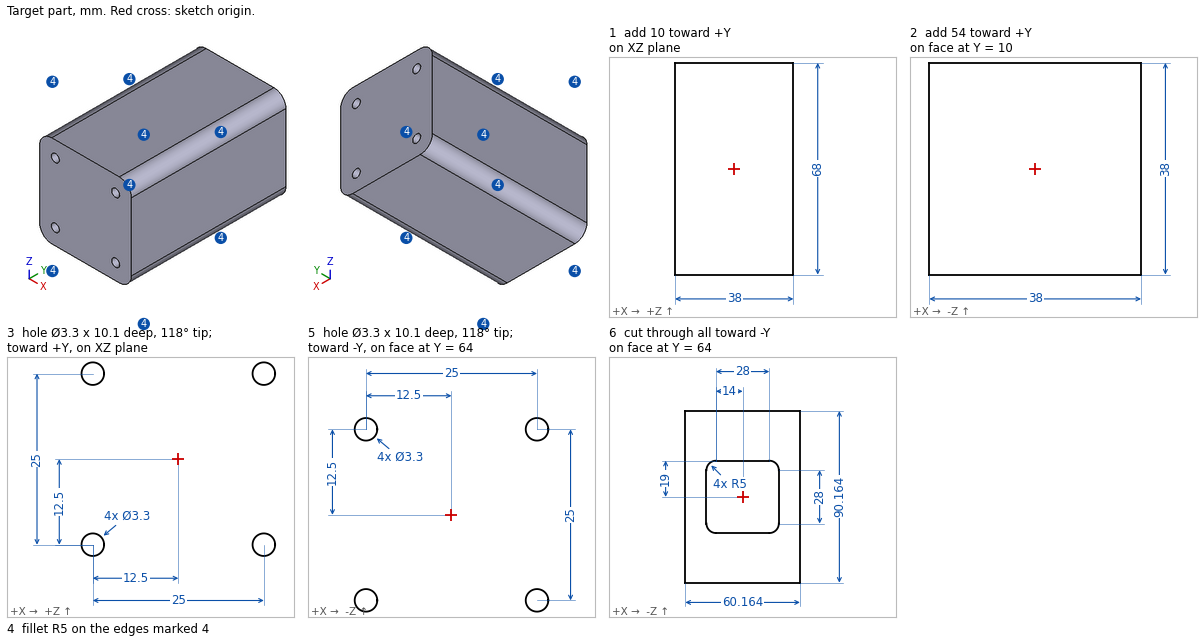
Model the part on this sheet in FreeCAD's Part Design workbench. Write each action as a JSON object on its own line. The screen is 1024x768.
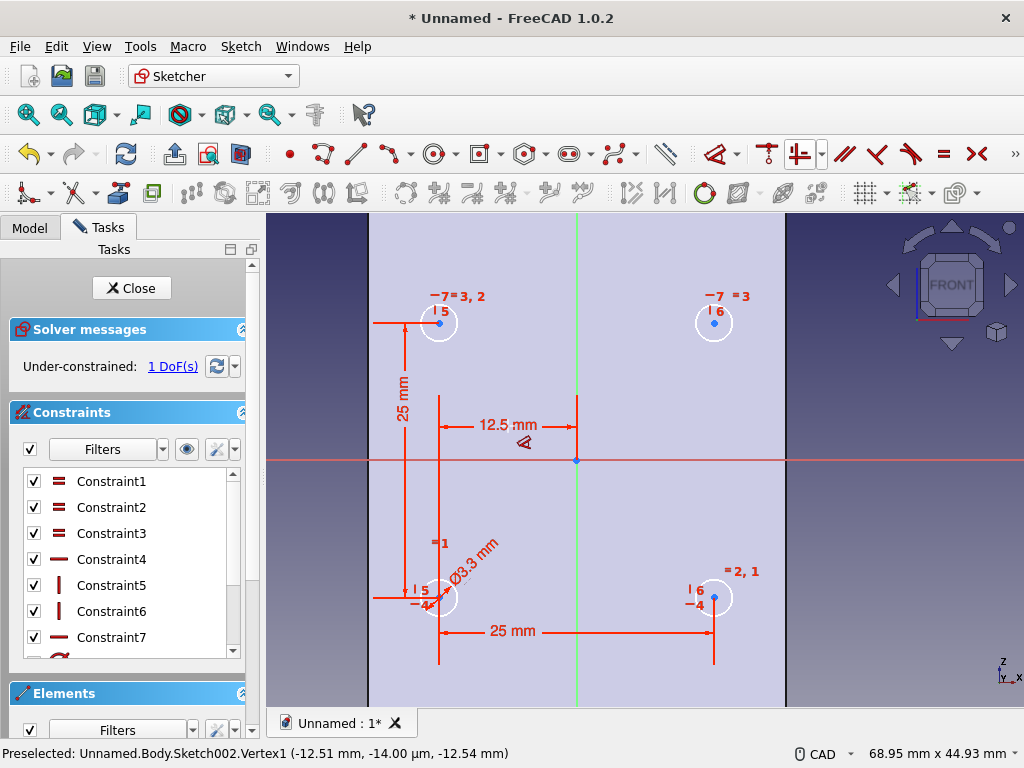
{"action": "left_click", "coordinate": [439, 598]}
{"action": "left_click", "coordinate": [405, 529]}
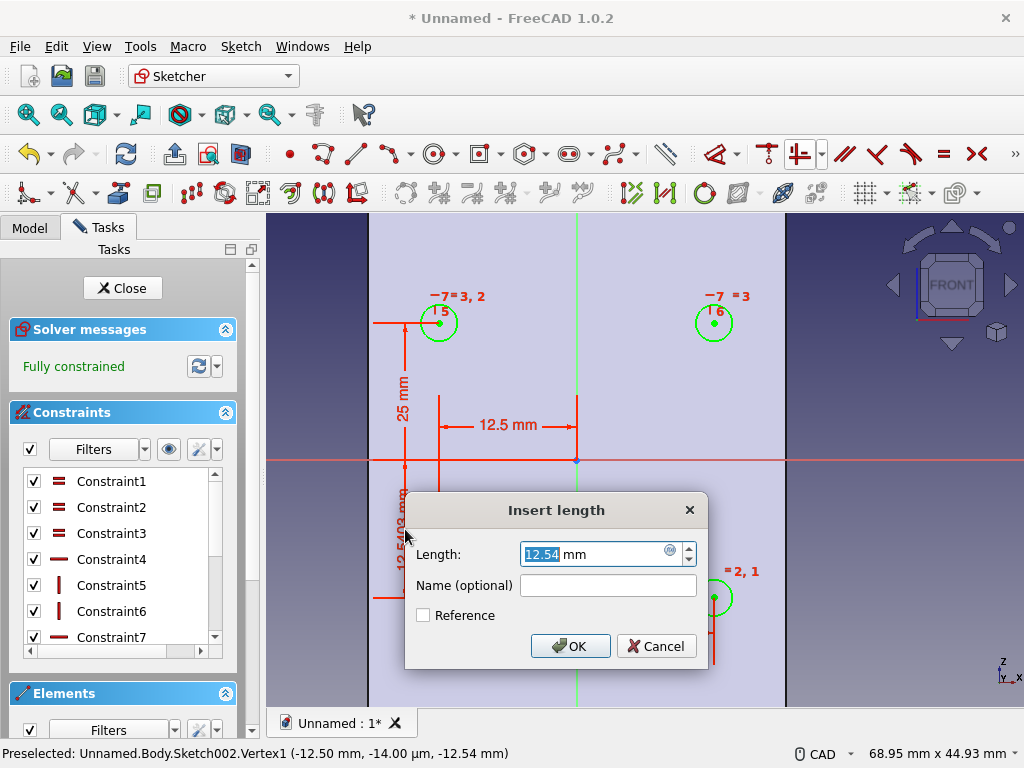
{"action": "type", "text": "12.5"}
{"action": "key", "text": "Return"}
{"action": "key", "text": "Escape"}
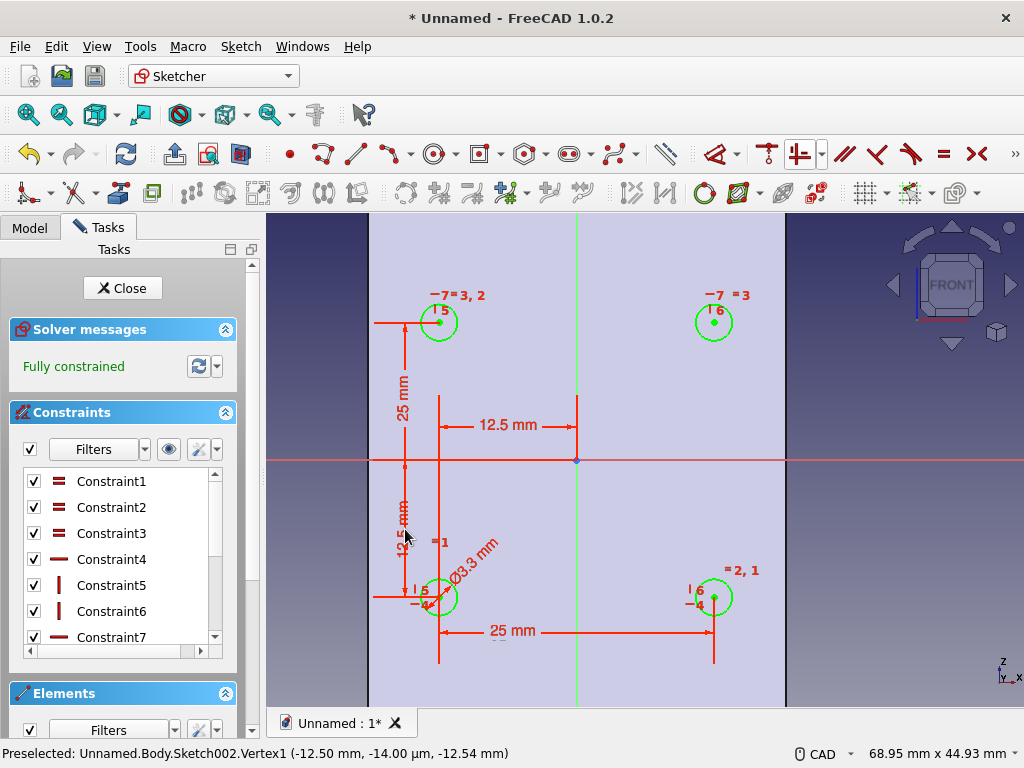
{"action": "left_click", "coordinate": [123, 288]}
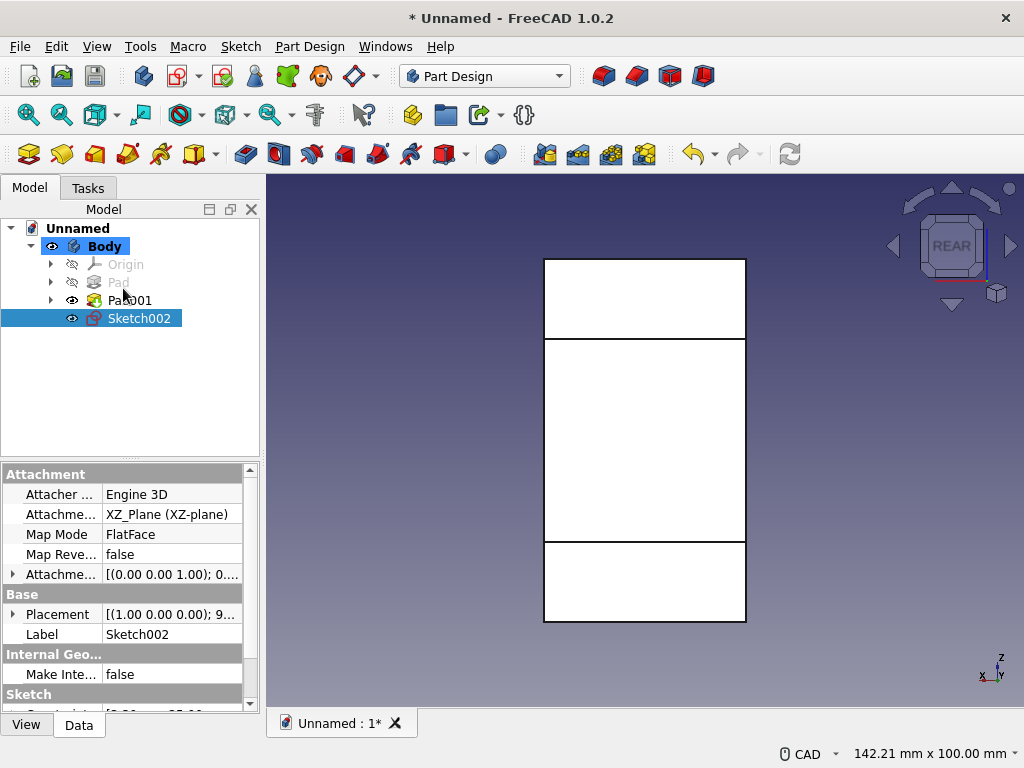
{"action": "left_click", "coordinate": [279, 154]}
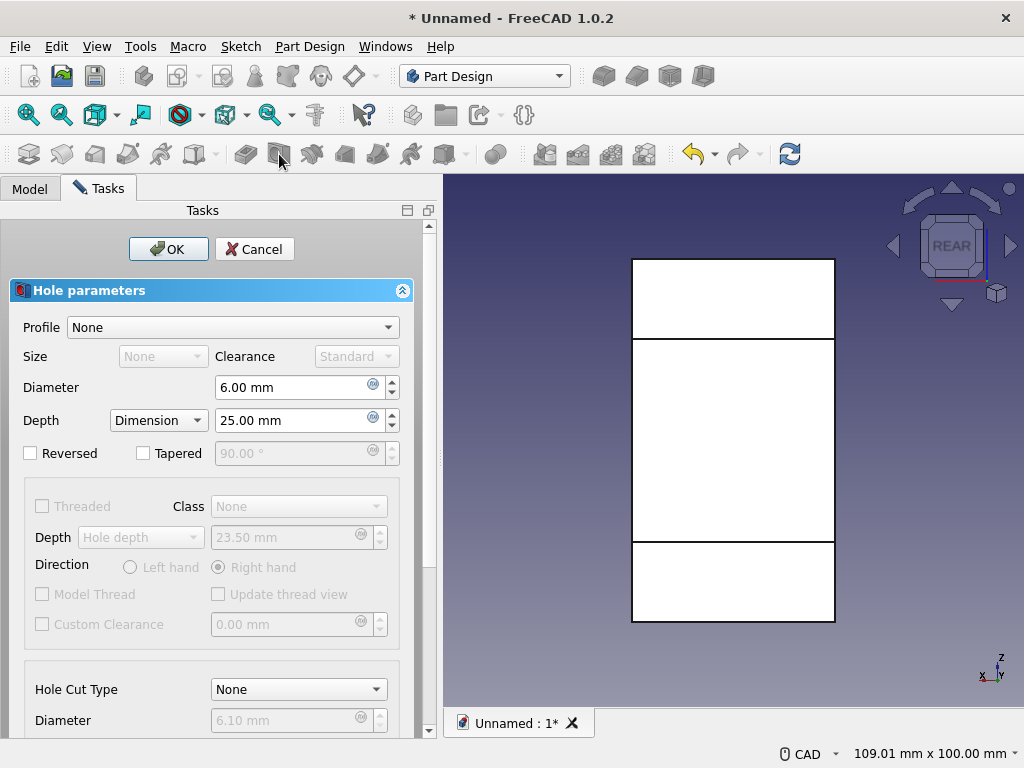
{"action": "triple_click", "coordinate": [300, 388]}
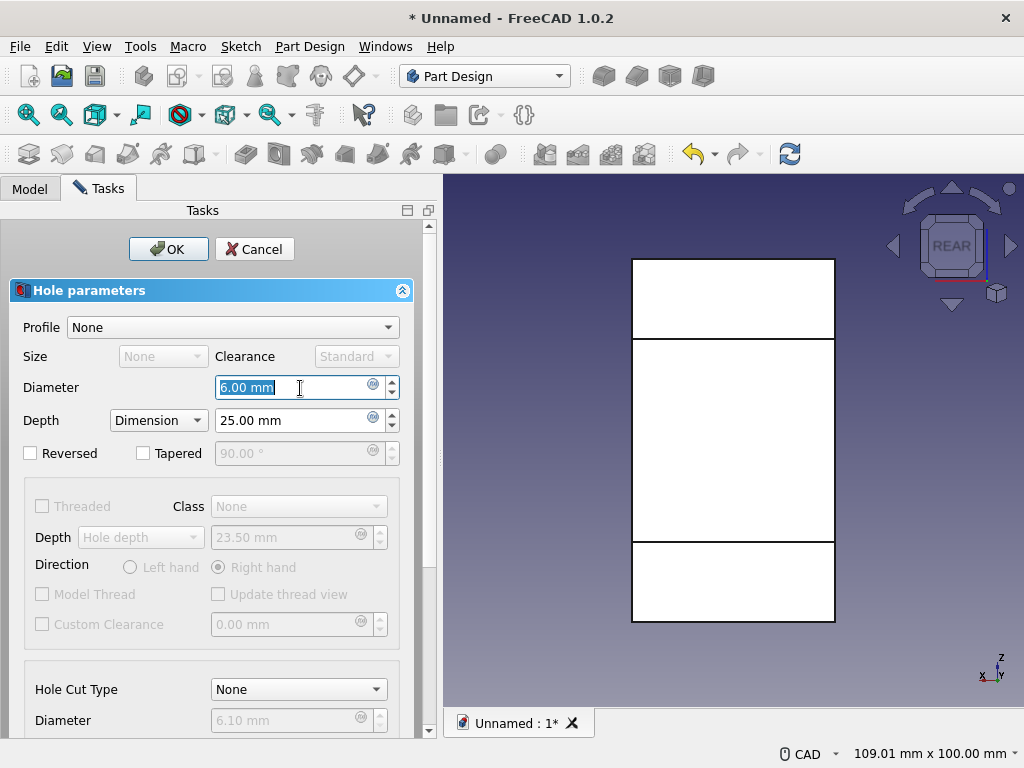
{"action": "type", "text": "3.3"}
{"action": "key", "text": "Tab"}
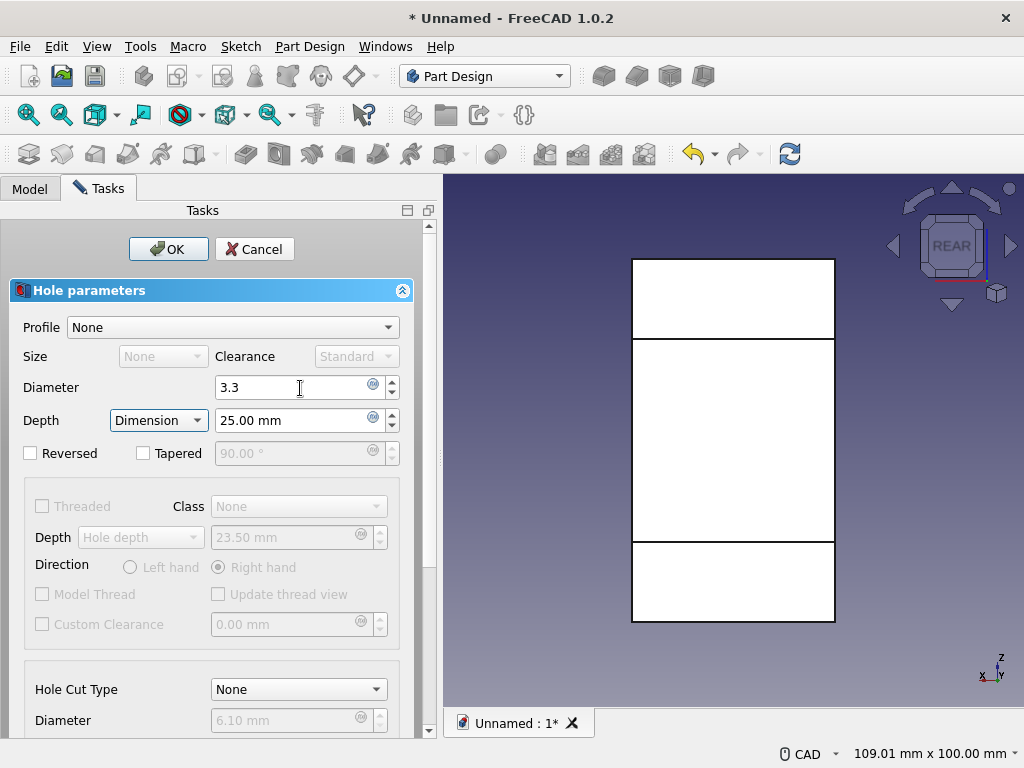
{"action": "triple_click", "coordinate": [300, 420]}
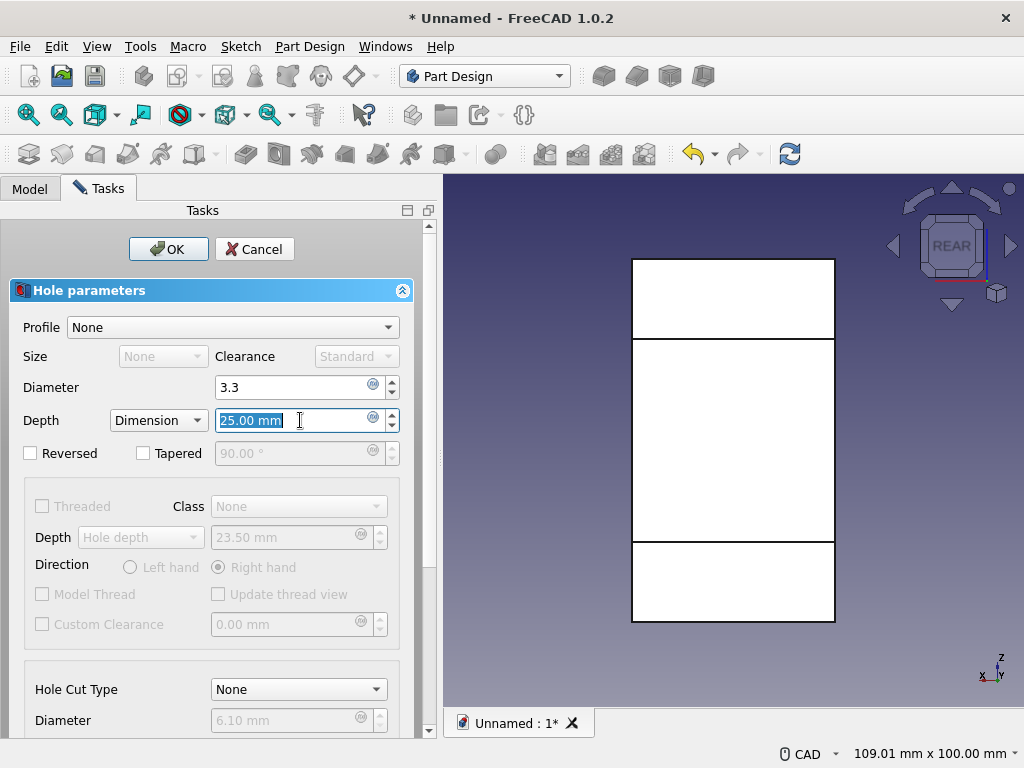
{"action": "type", "text": "10.1"}
{"action": "key", "text": "Tab"}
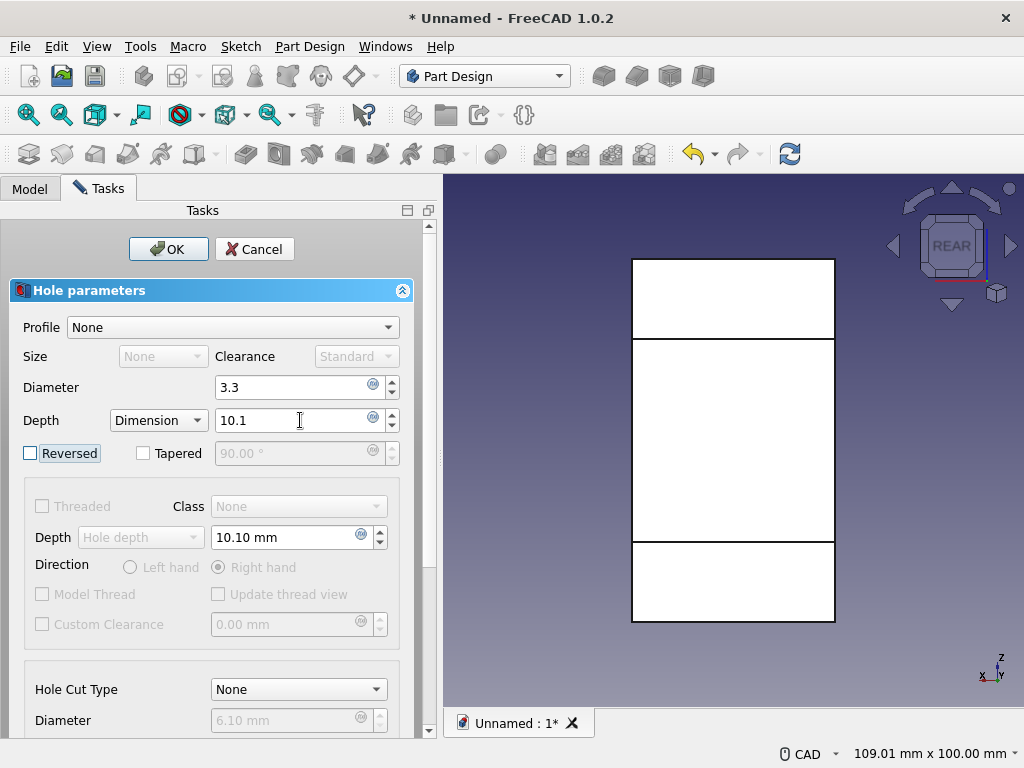
{"action": "left_click", "coordinate": [169, 249]}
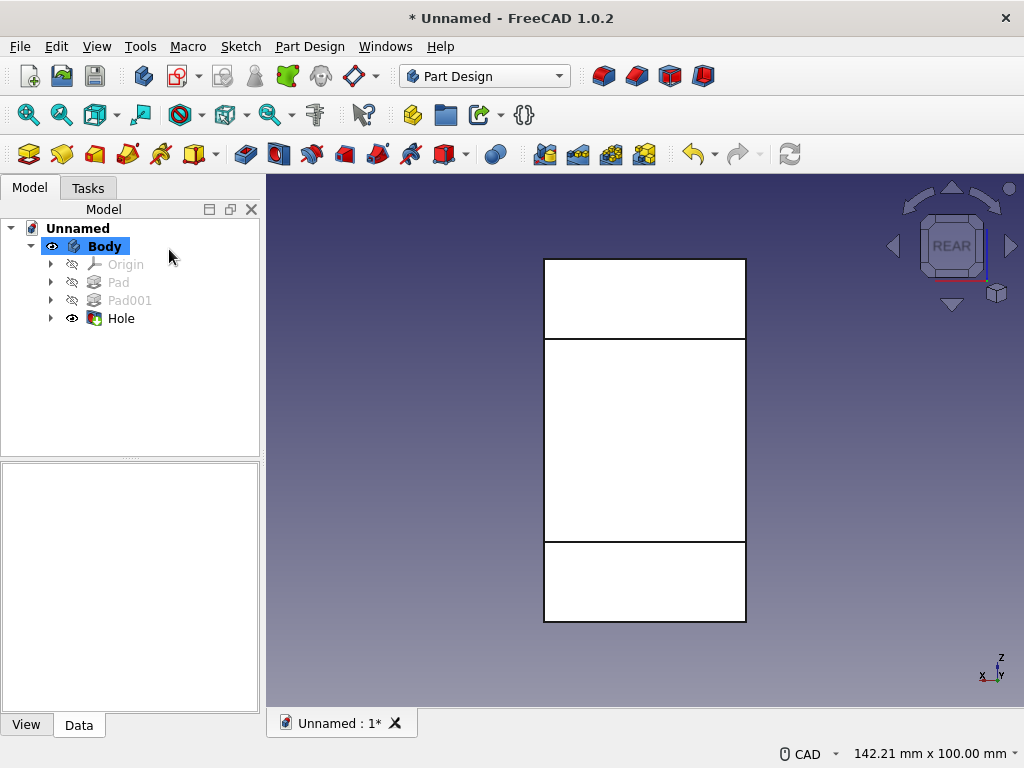
{"action": "key", "text": "0"}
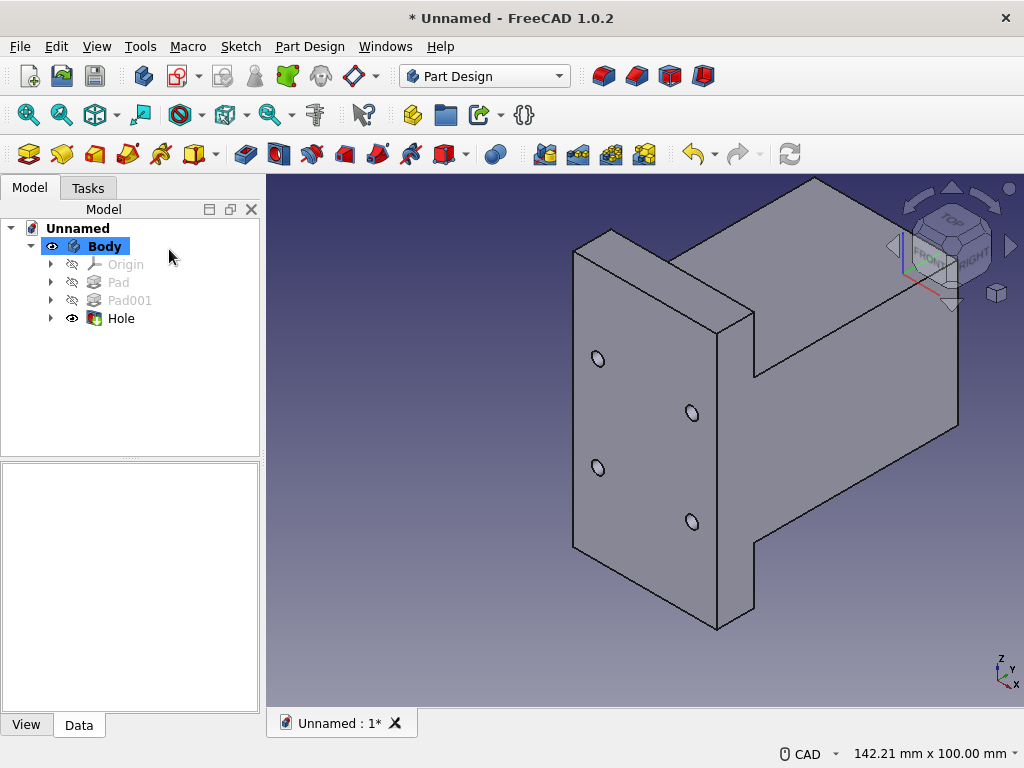
{"action": "left_click", "coordinate": [29, 116]}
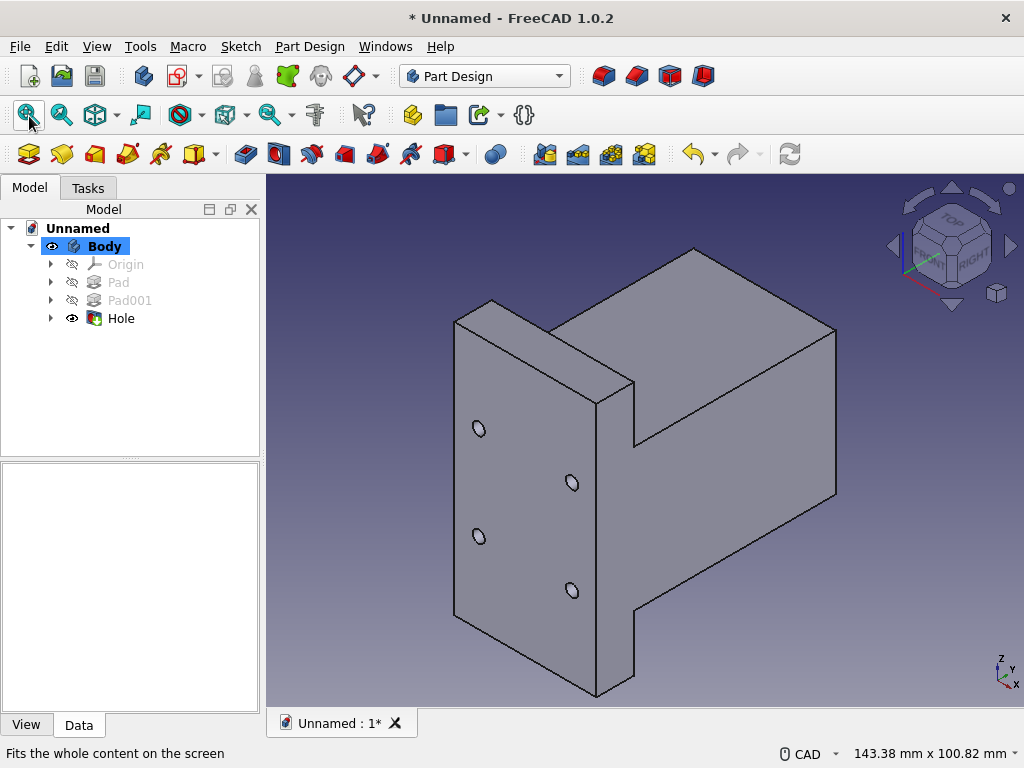
{"action": "left_click", "coordinate": [735, 388]}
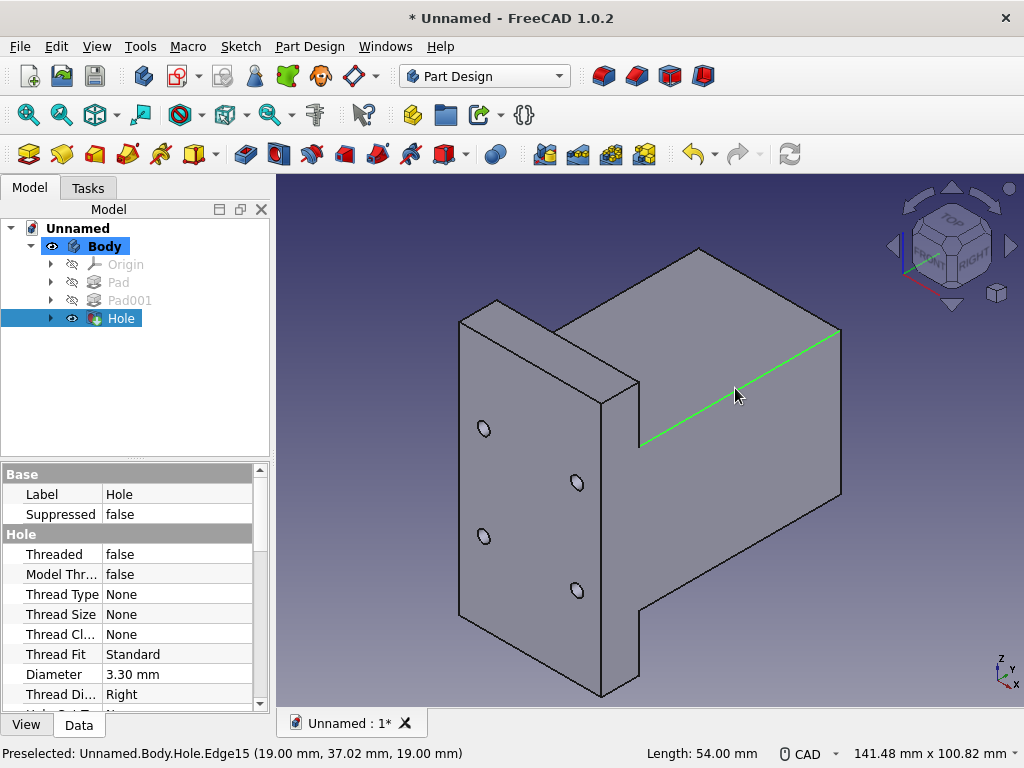
{"action": "left_click", "coordinate": [620, 392], "text": "ctrl"}